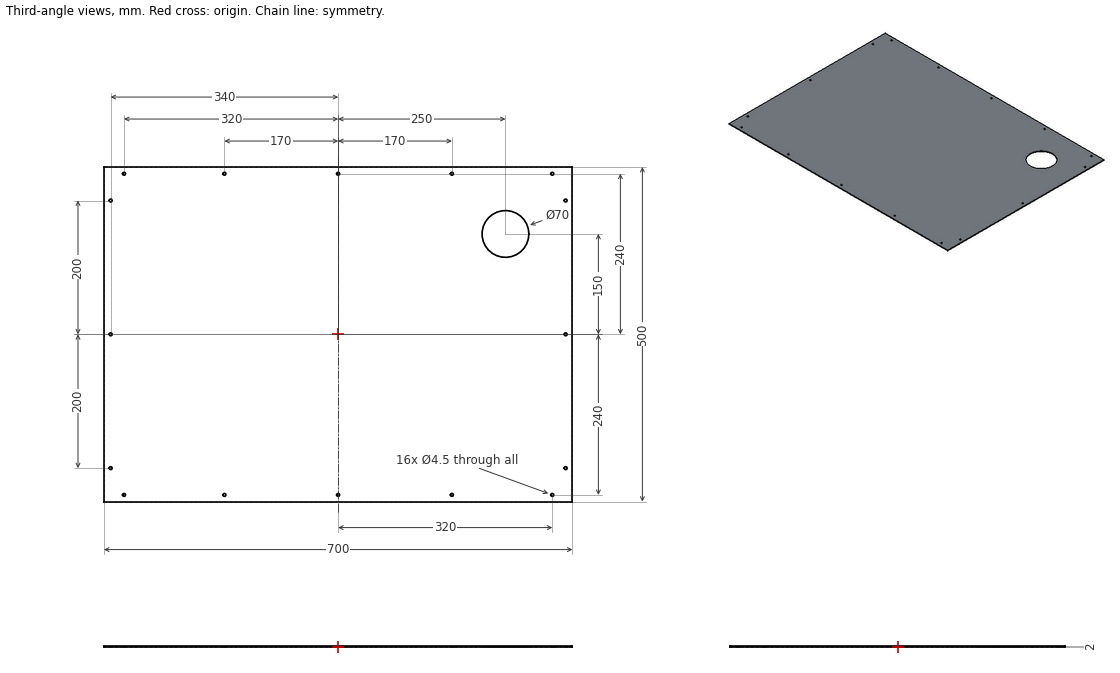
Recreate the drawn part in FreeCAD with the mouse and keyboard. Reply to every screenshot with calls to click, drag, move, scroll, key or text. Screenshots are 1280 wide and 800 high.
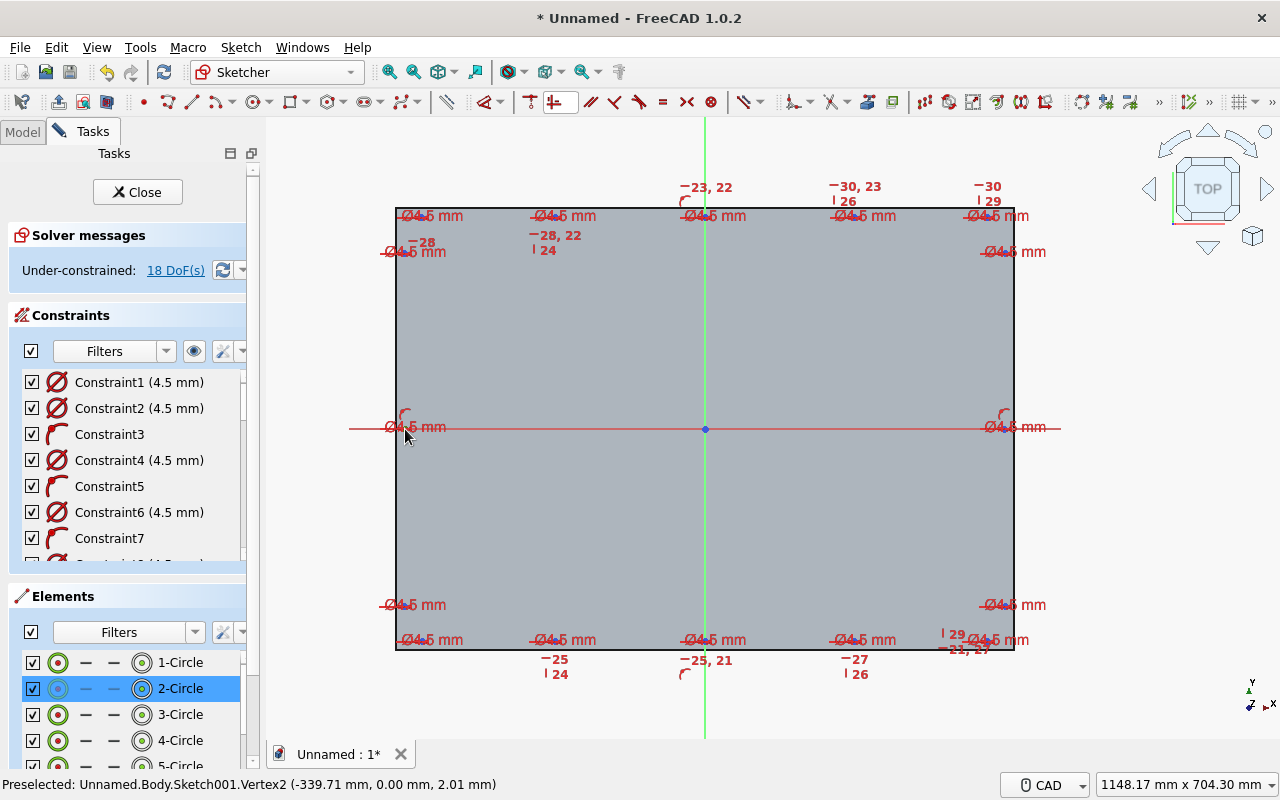
click(405, 254)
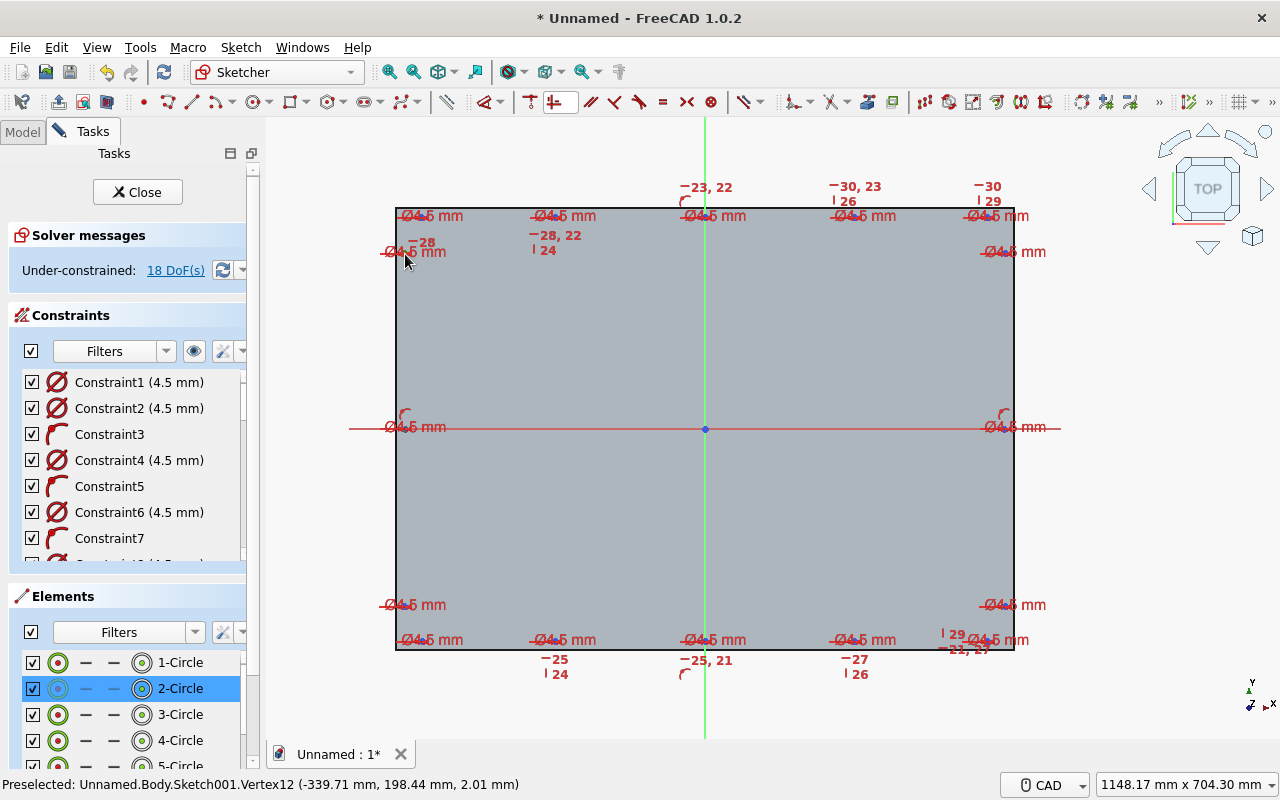
key(v)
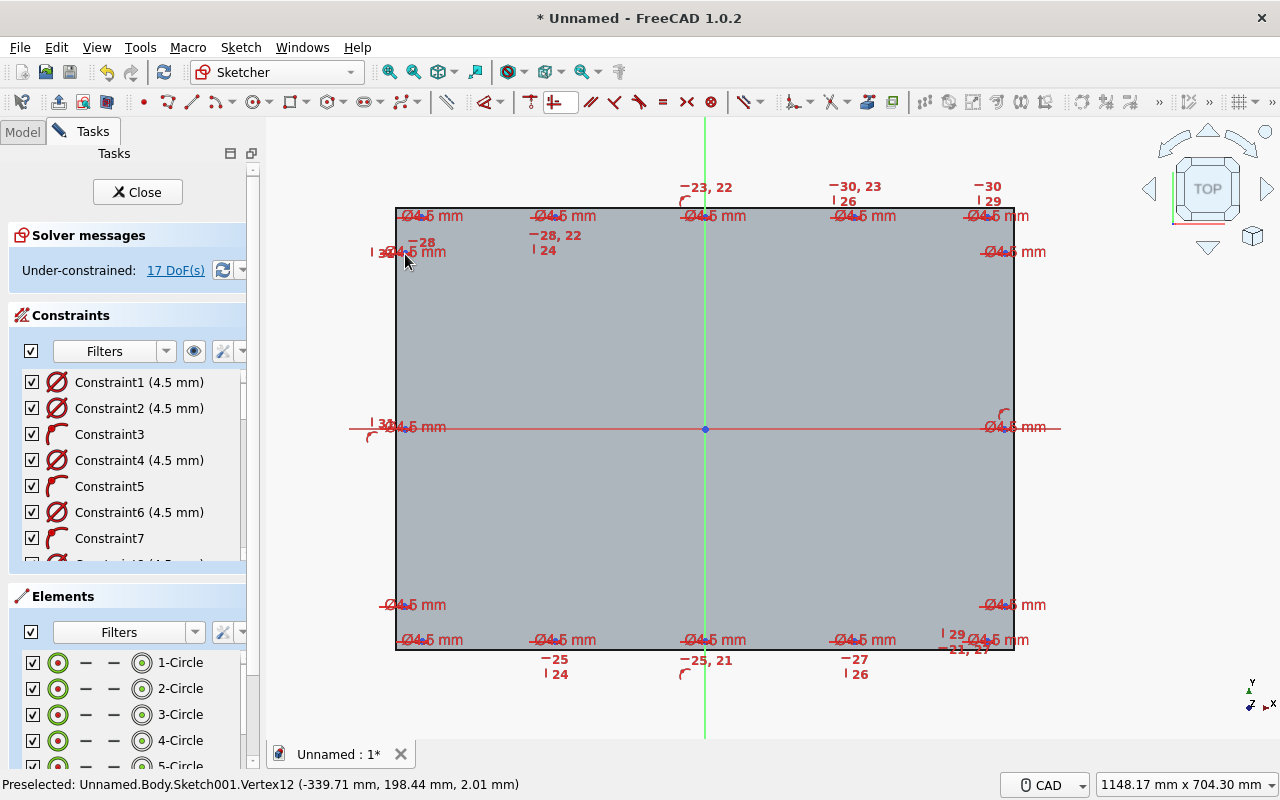
click(405, 429)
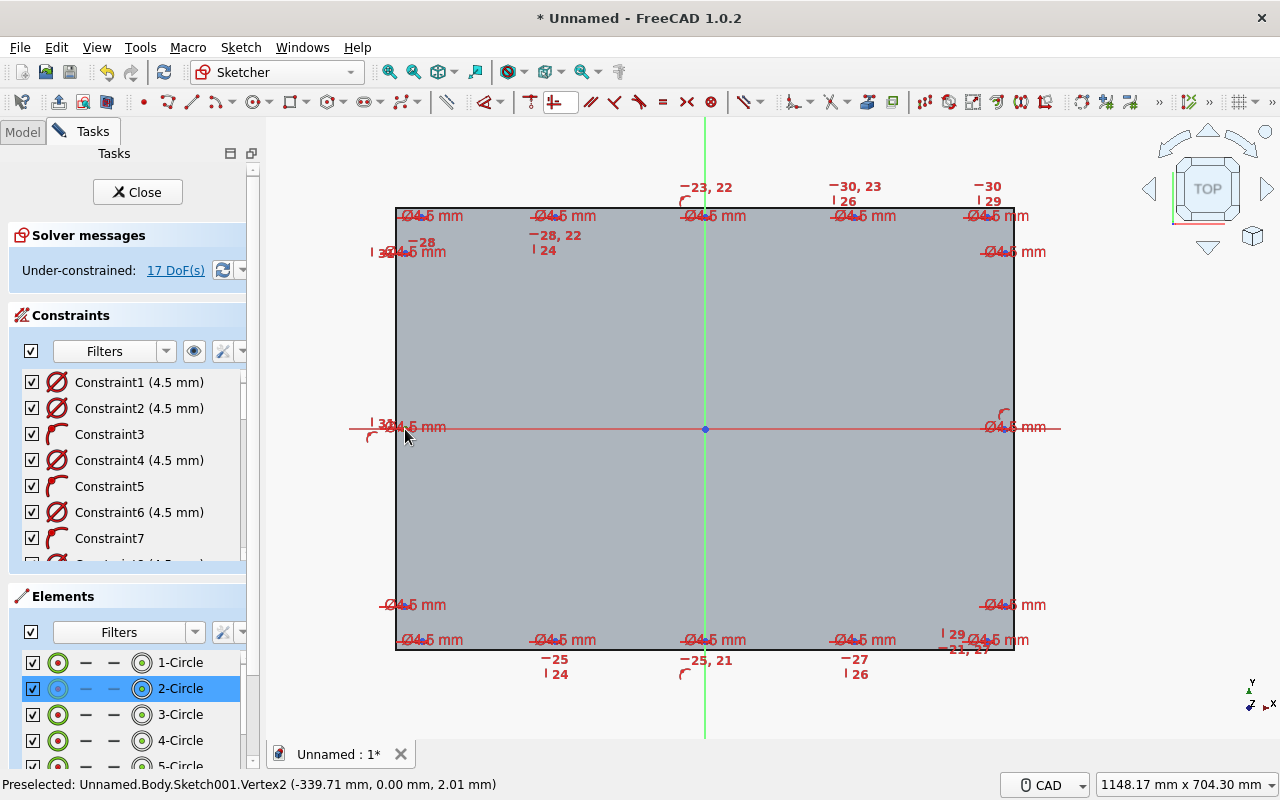
click(405, 607)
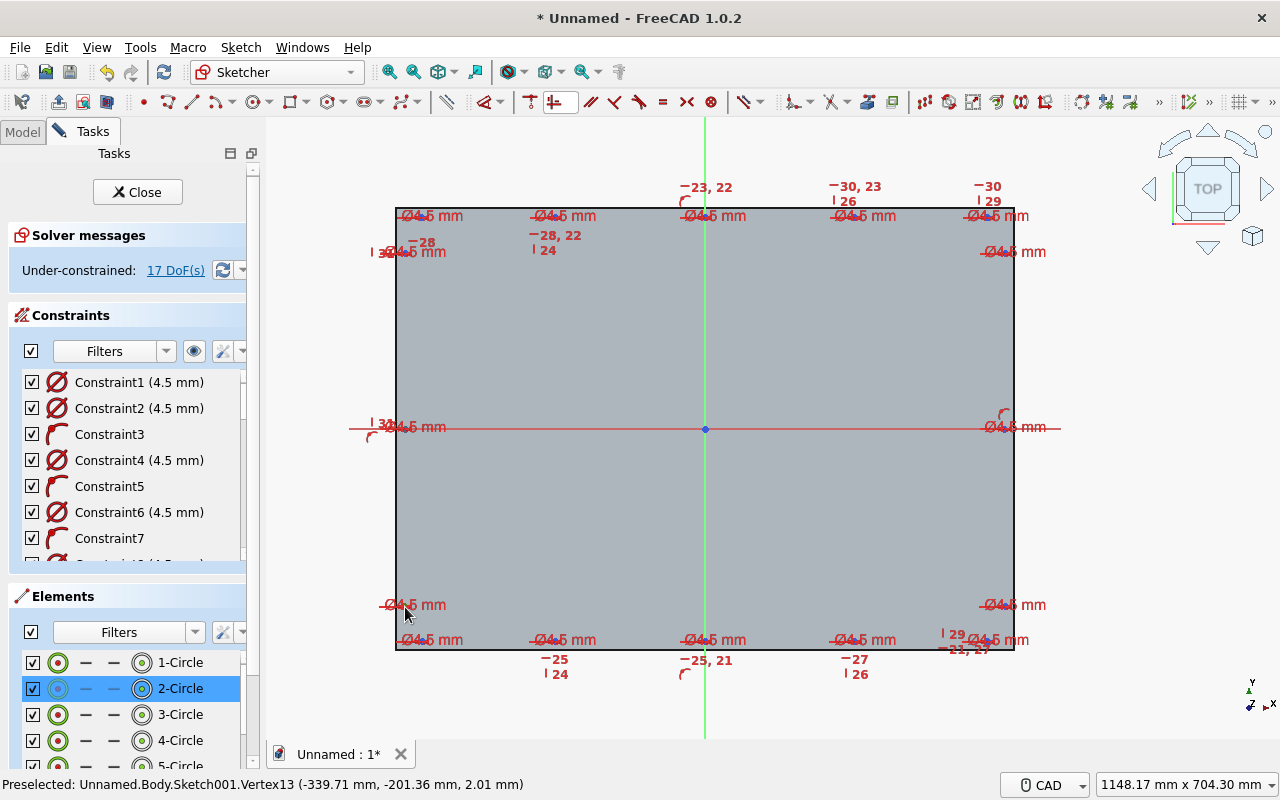
click(572, 102)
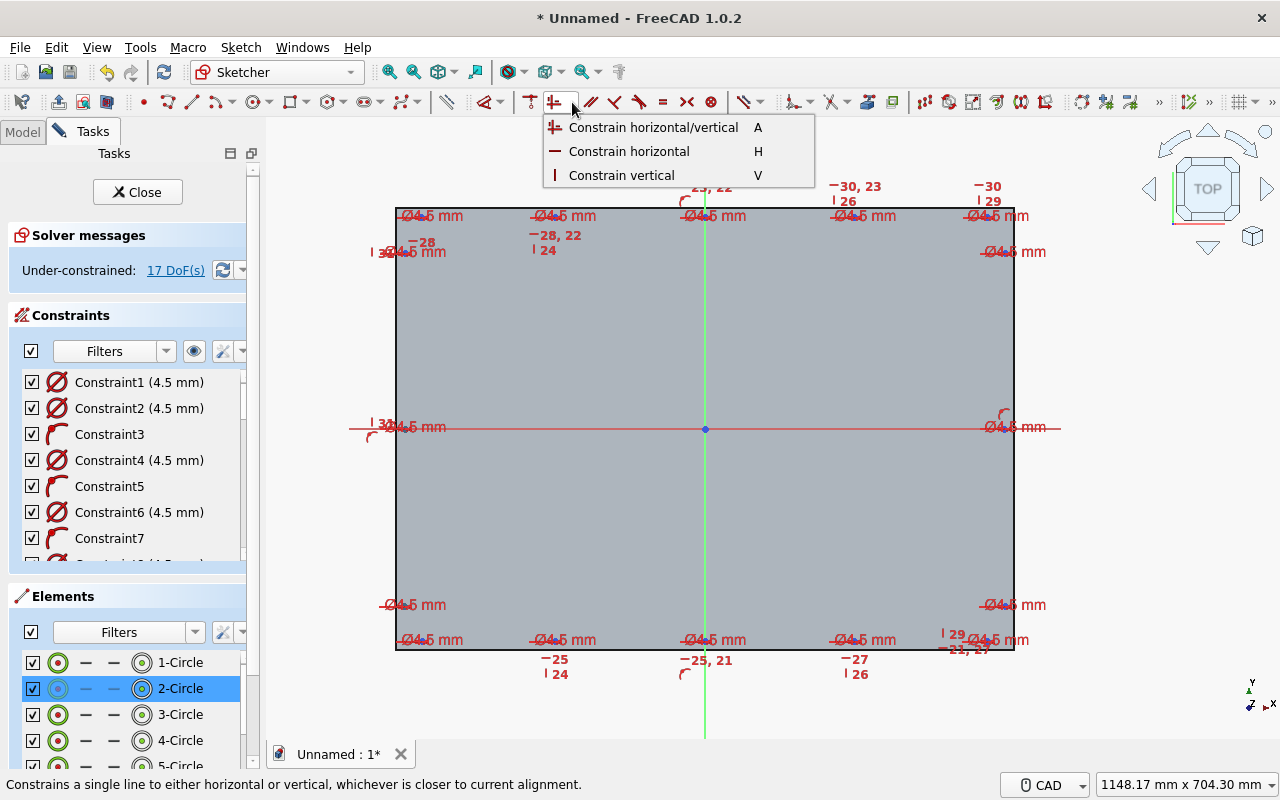
click(679, 175)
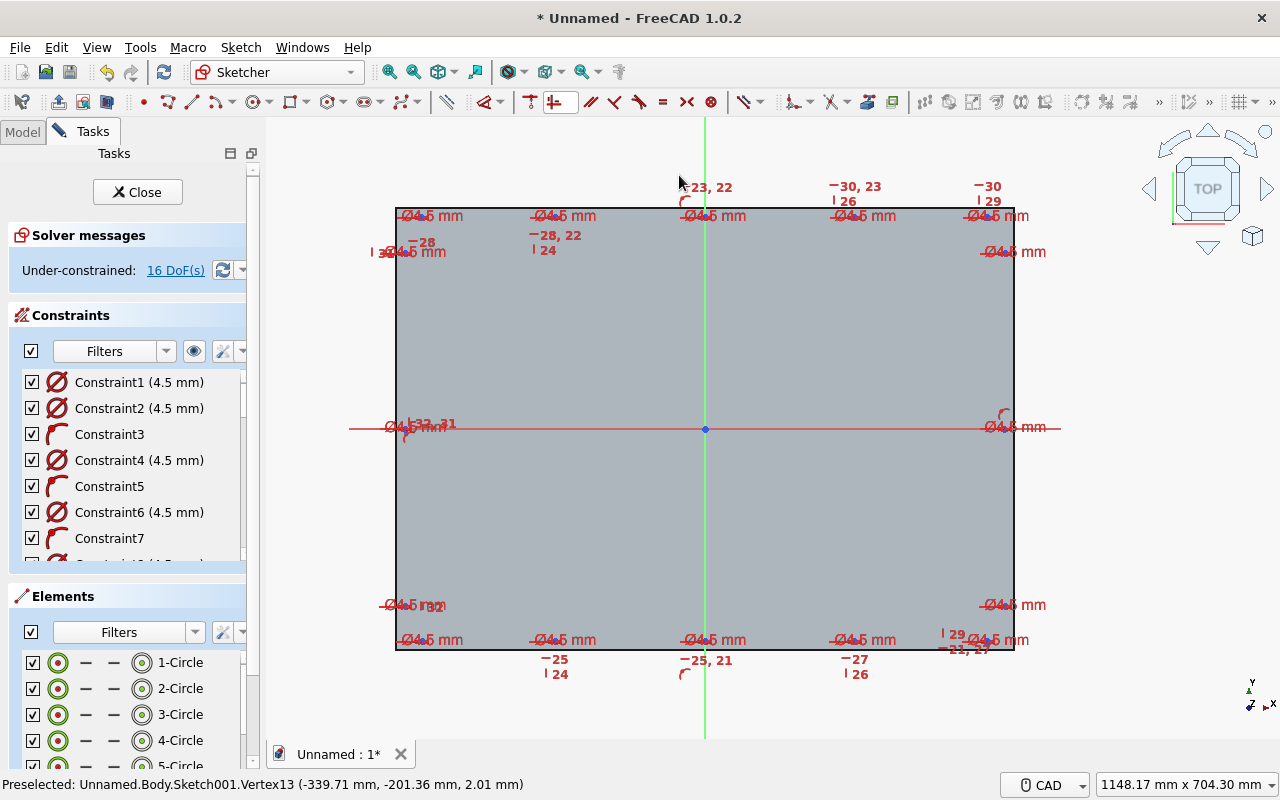
click(1005, 429)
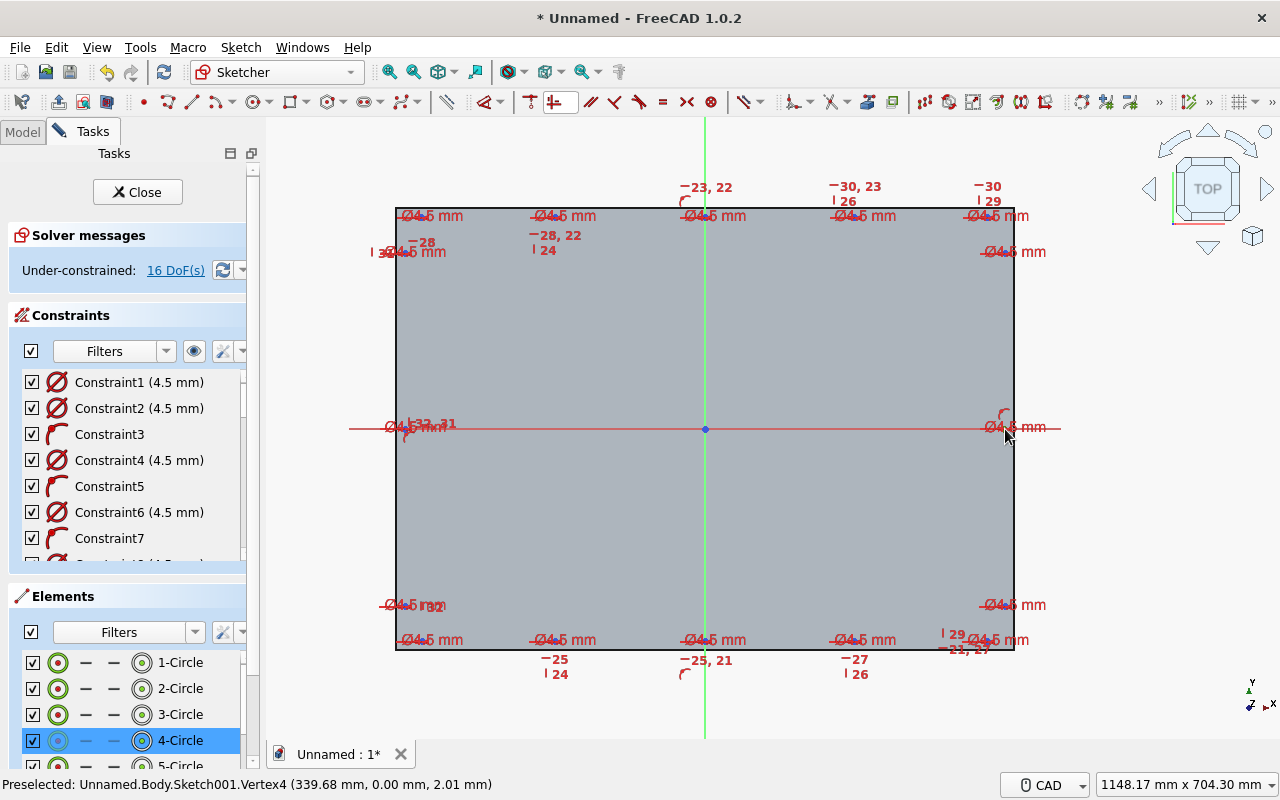
click(1005, 607)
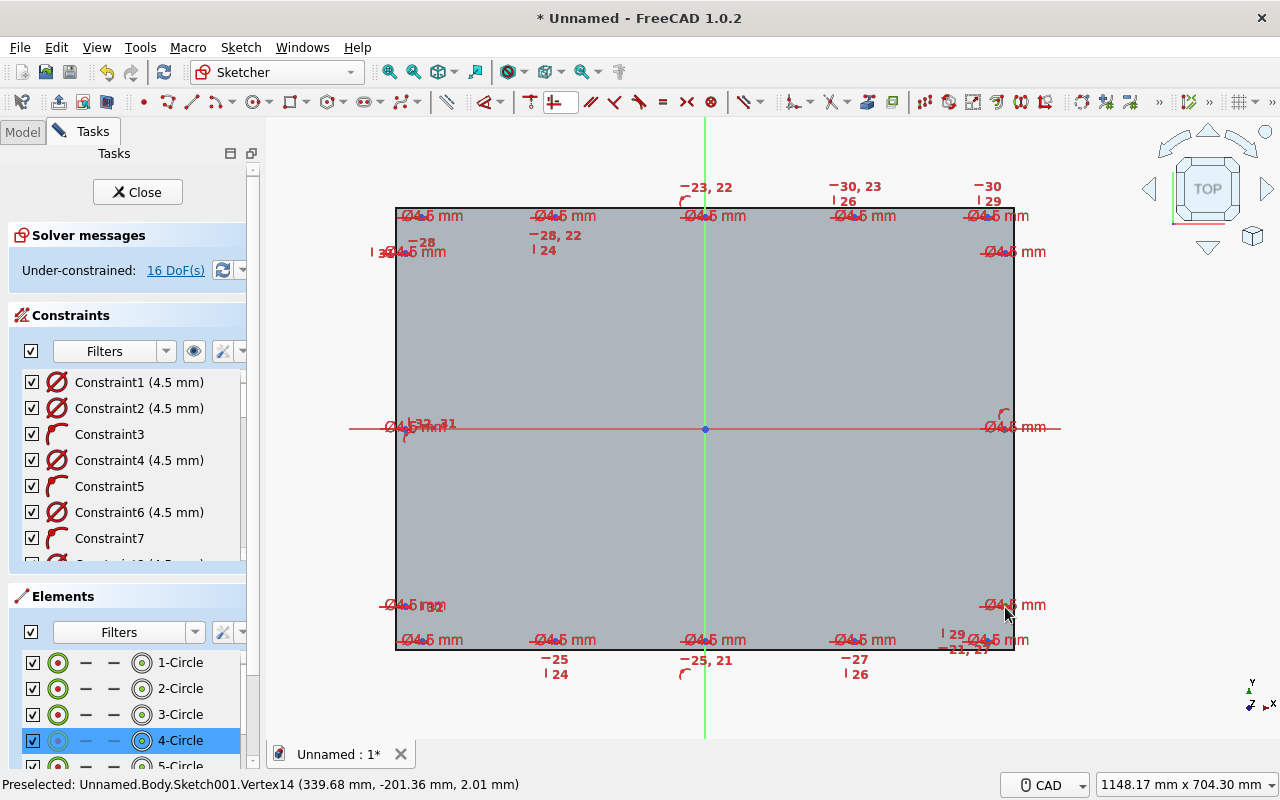
key(v)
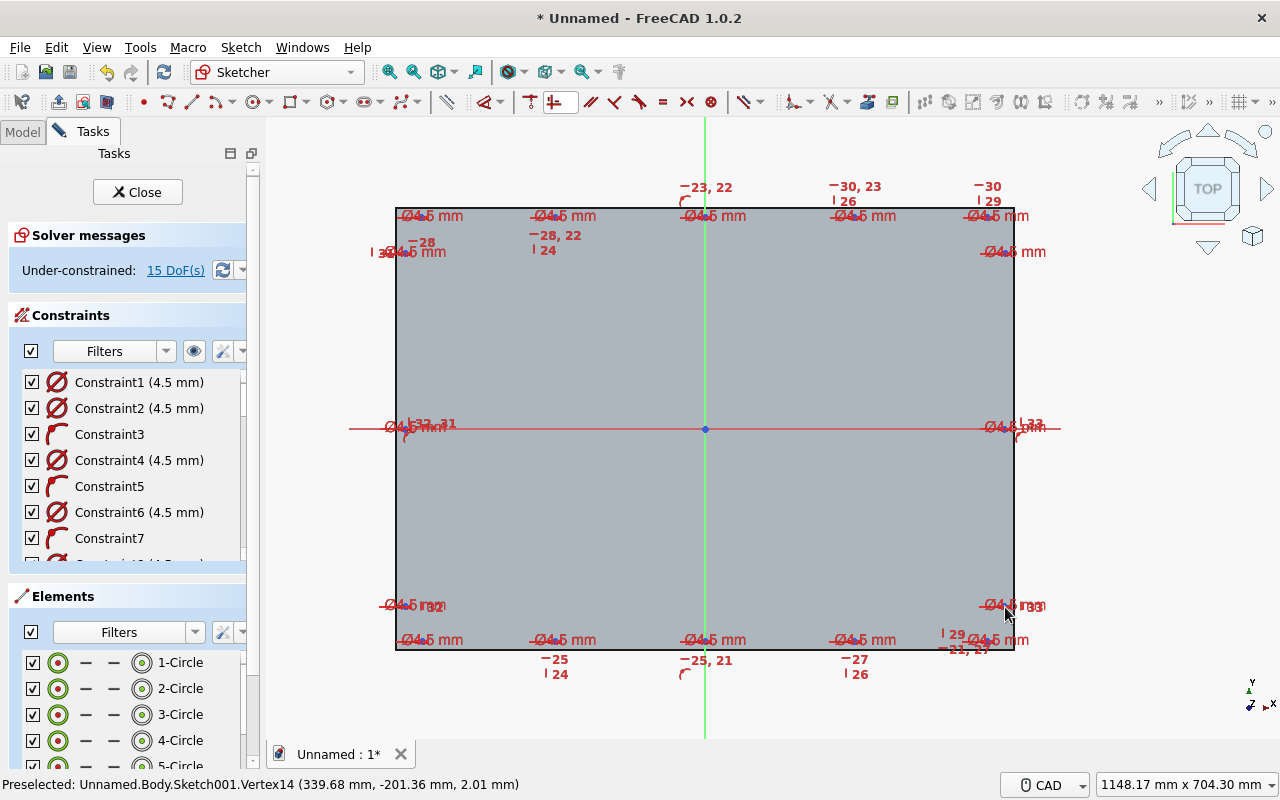
click(1005, 429)